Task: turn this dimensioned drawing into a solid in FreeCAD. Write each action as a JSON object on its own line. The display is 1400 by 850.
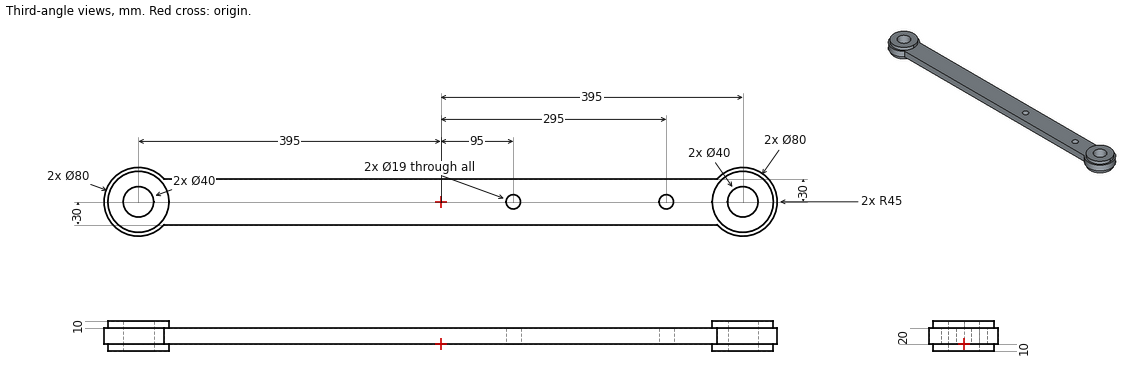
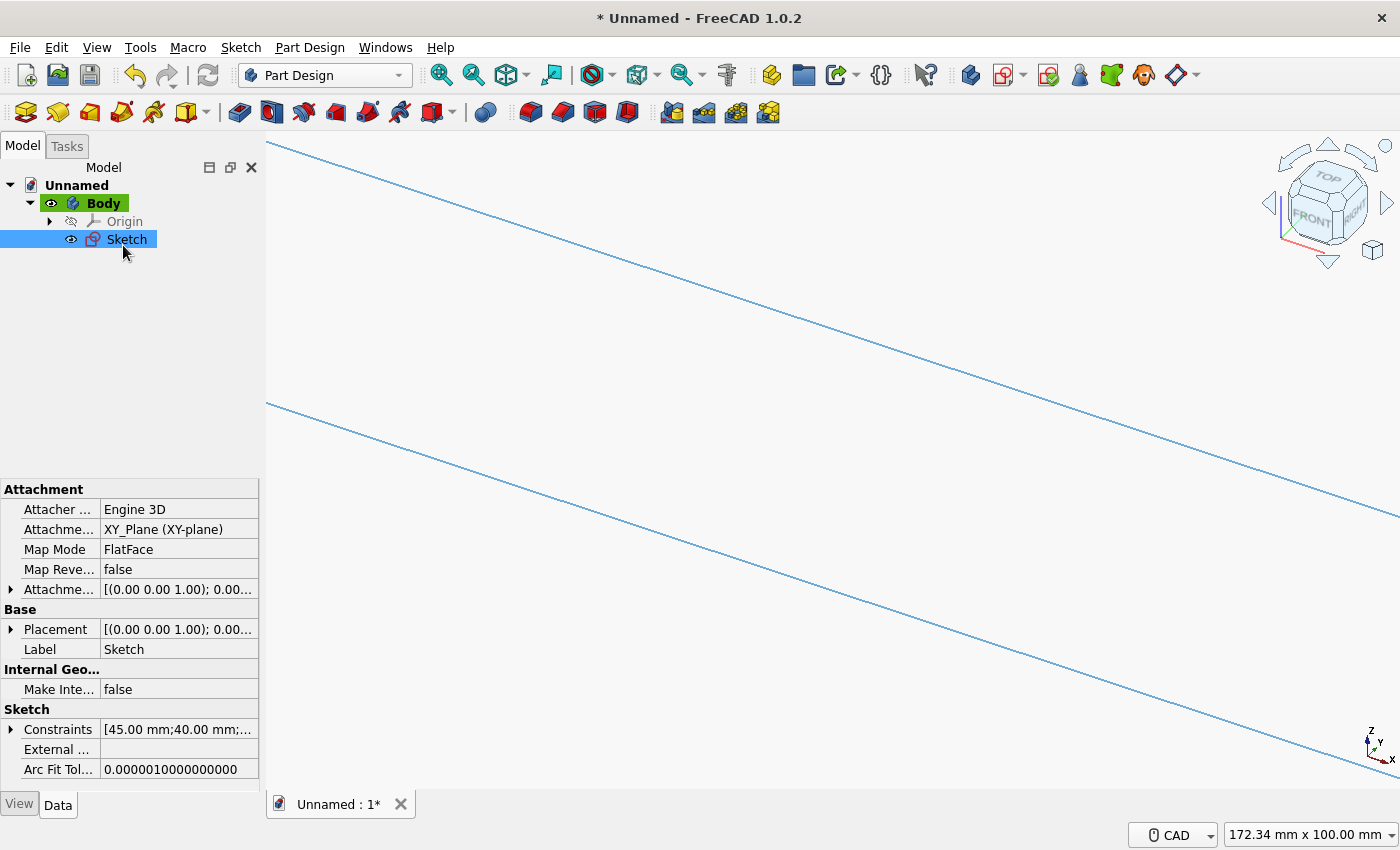
{"action": "left_click", "coordinate": [26, 112]}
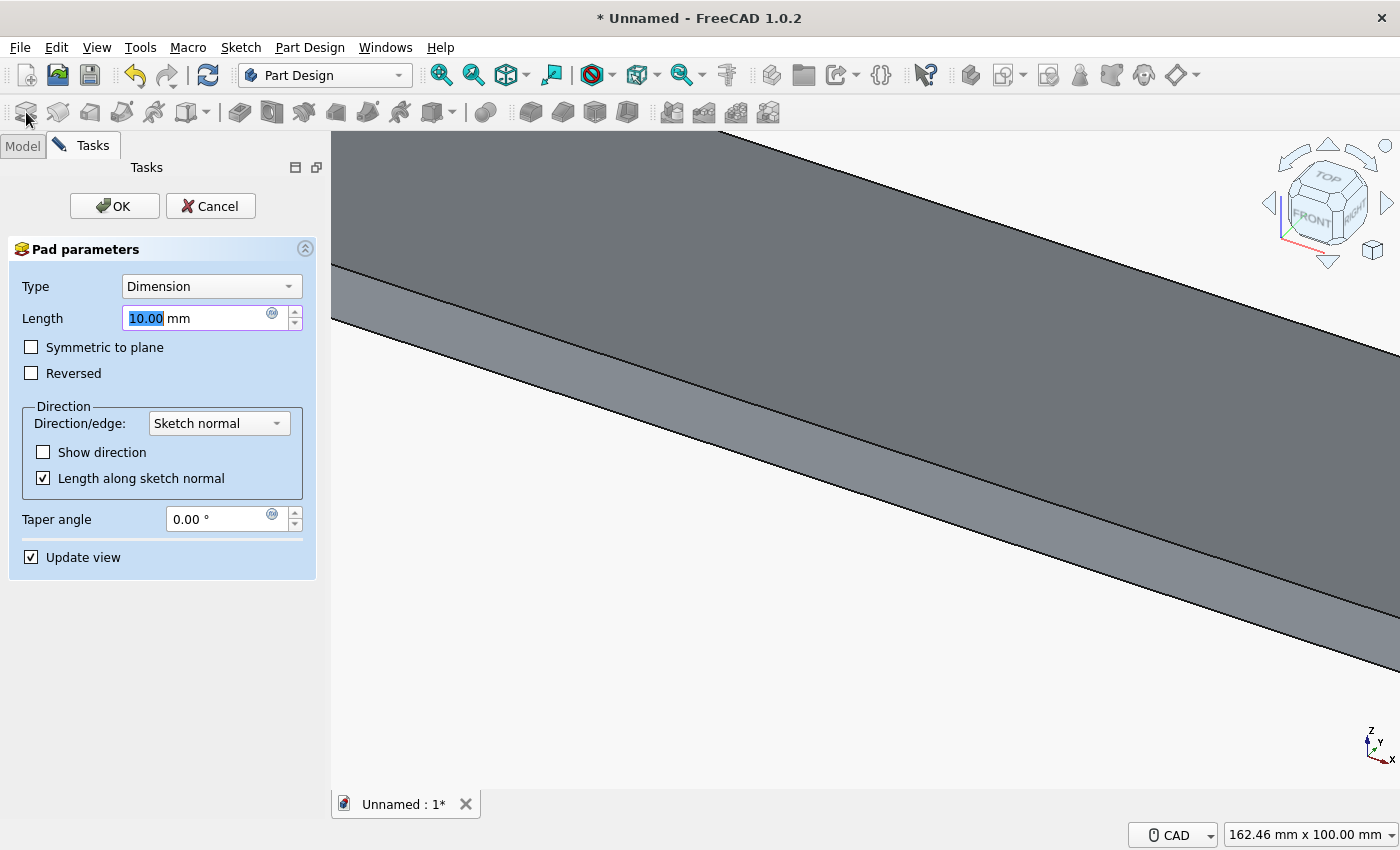
{"action": "type", "text": "20"}
{"action": "key", "text": "Tab"}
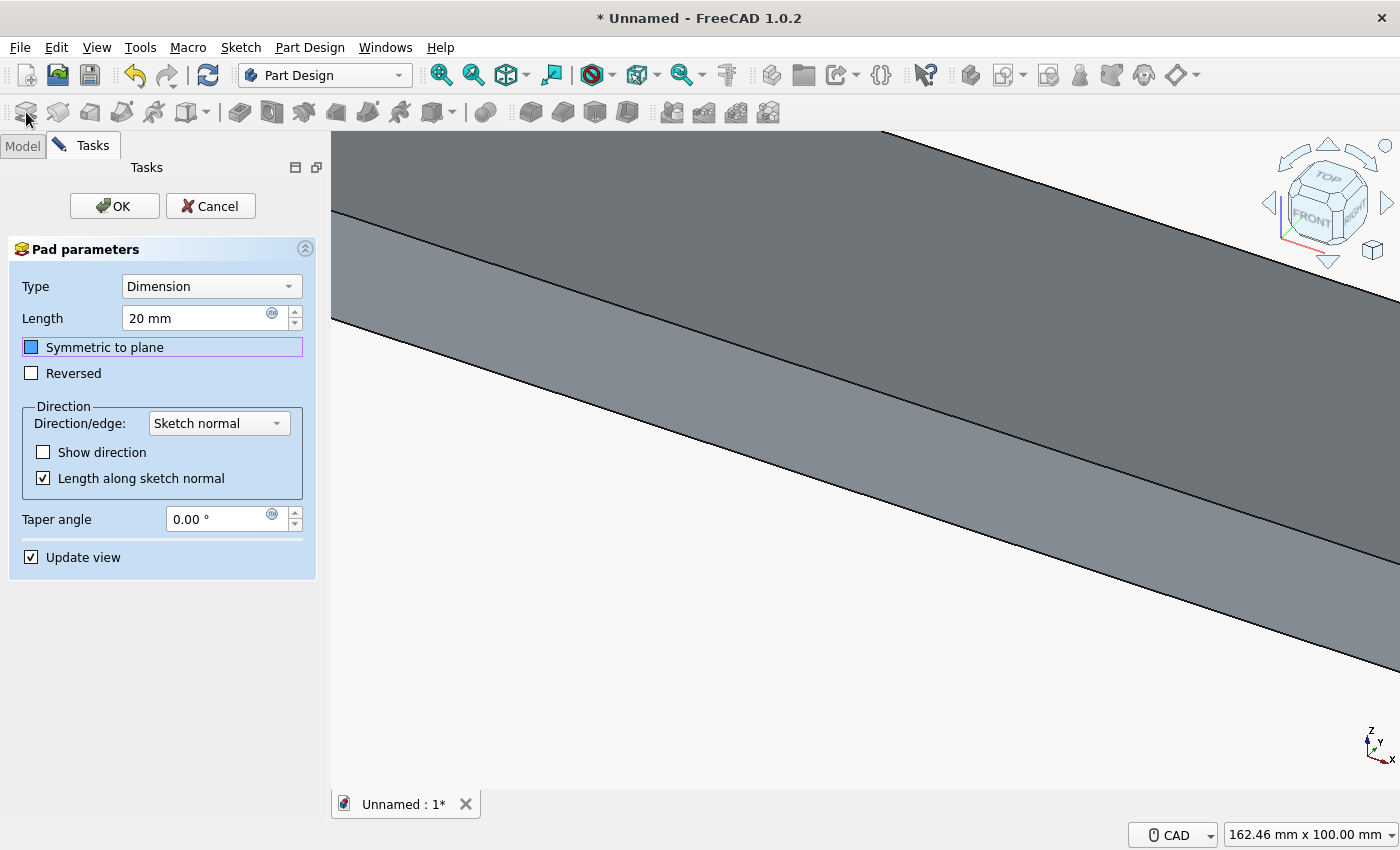
{"action": "left_click", "coordinate": [115, 206]}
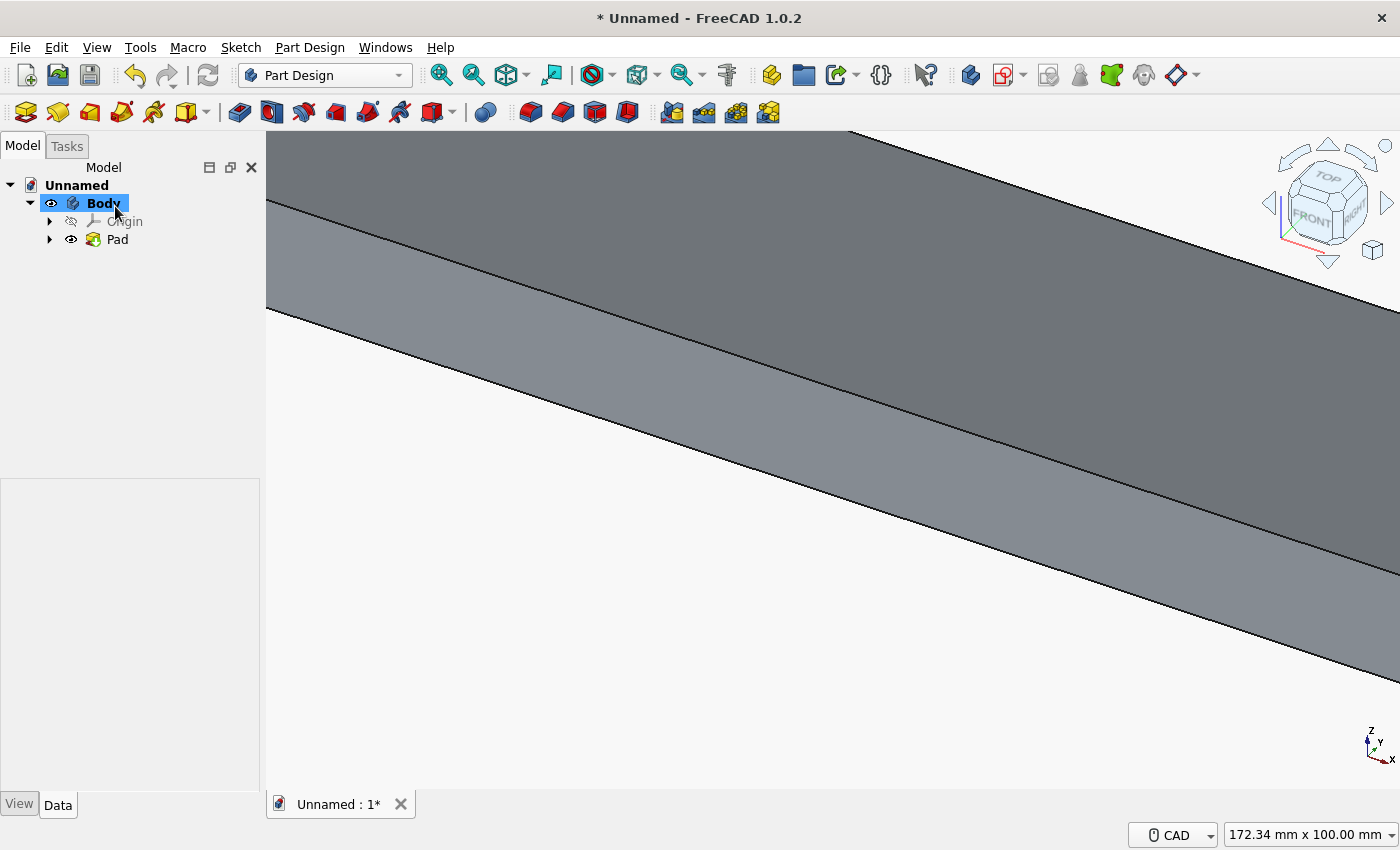
{"action": "left_click", "coordinate": [442, 76]}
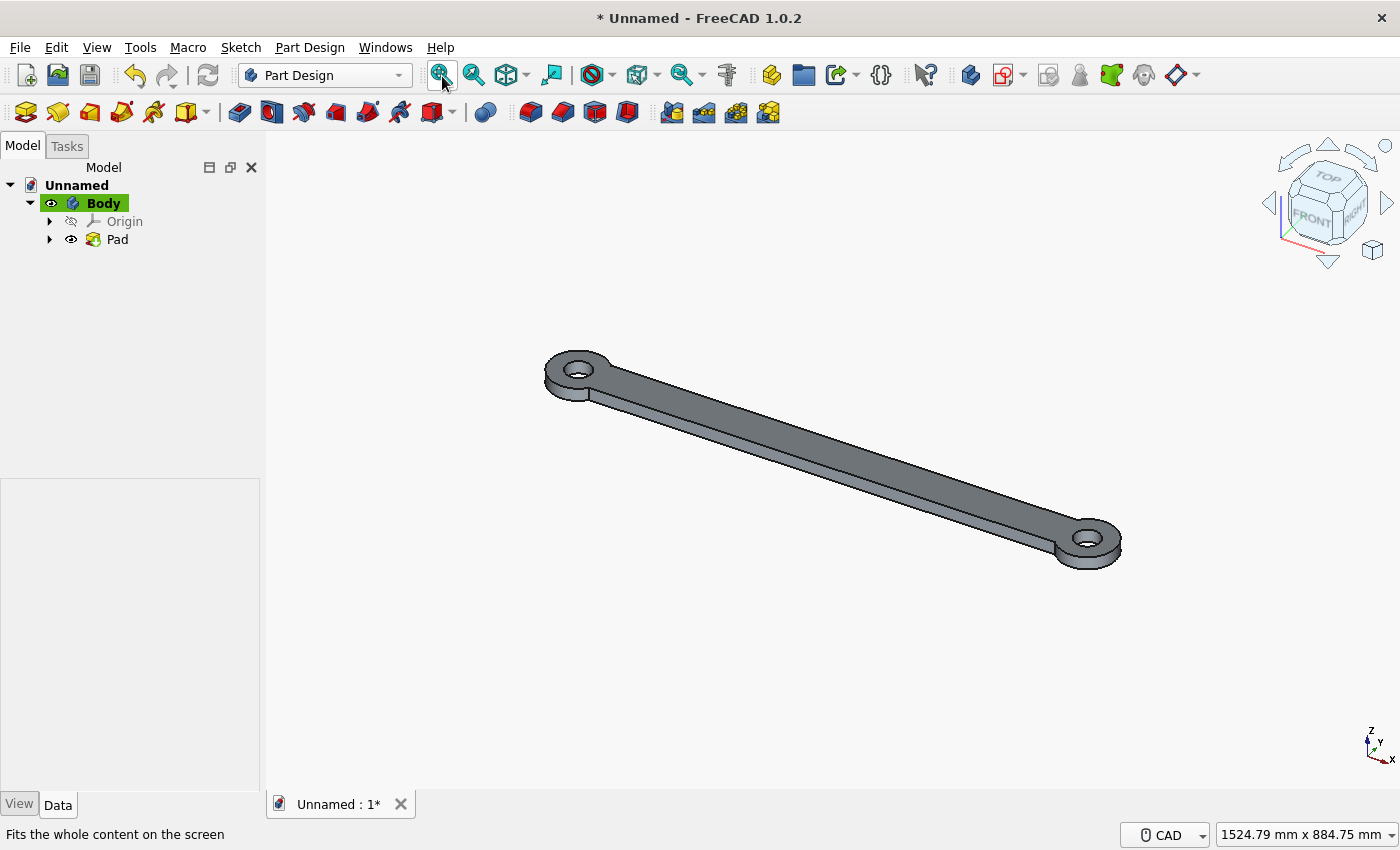
{"action": "left_click", "coordinate": [995, 507]}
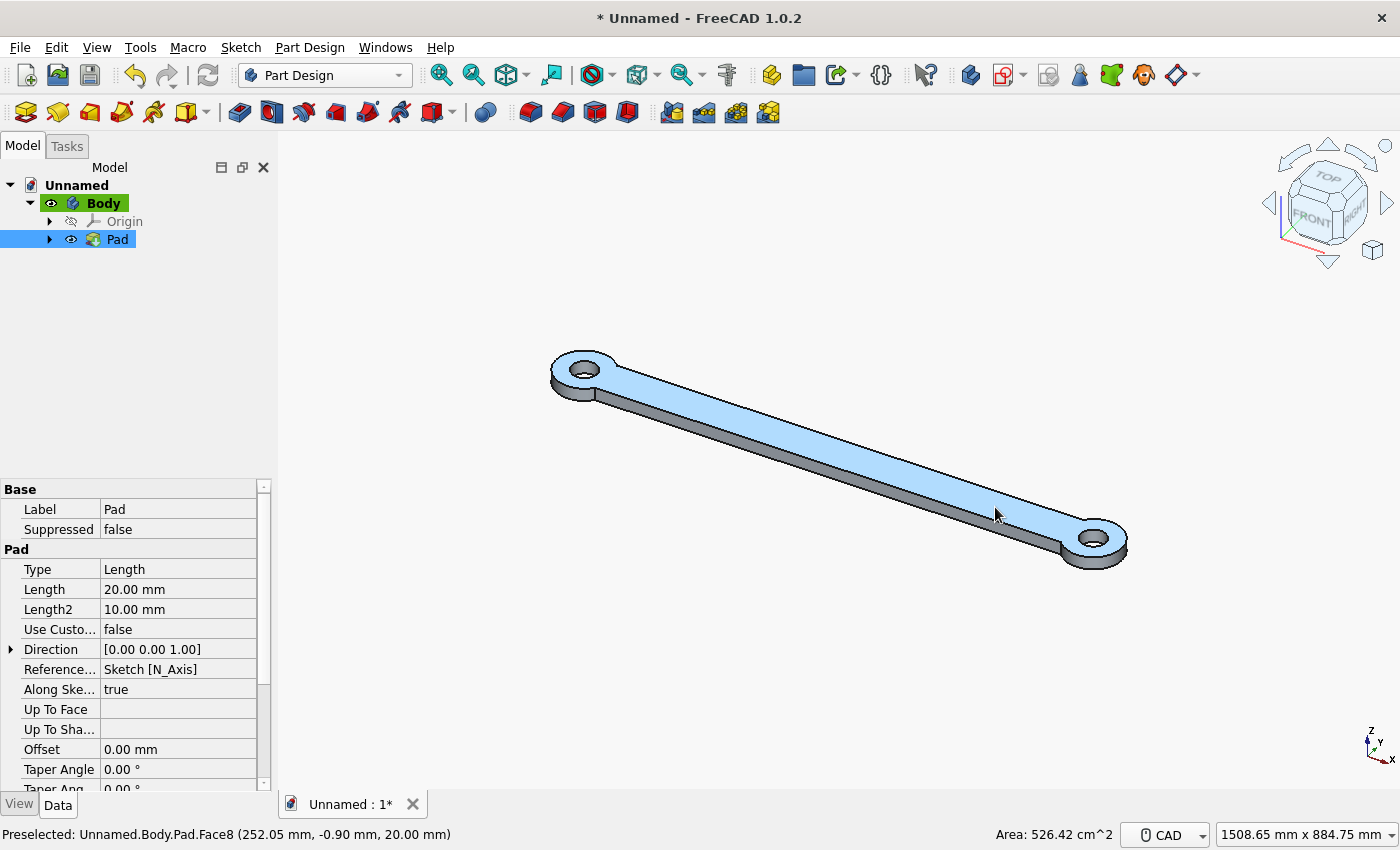
{"action": "left_click", "coordinate": [1004, 76]}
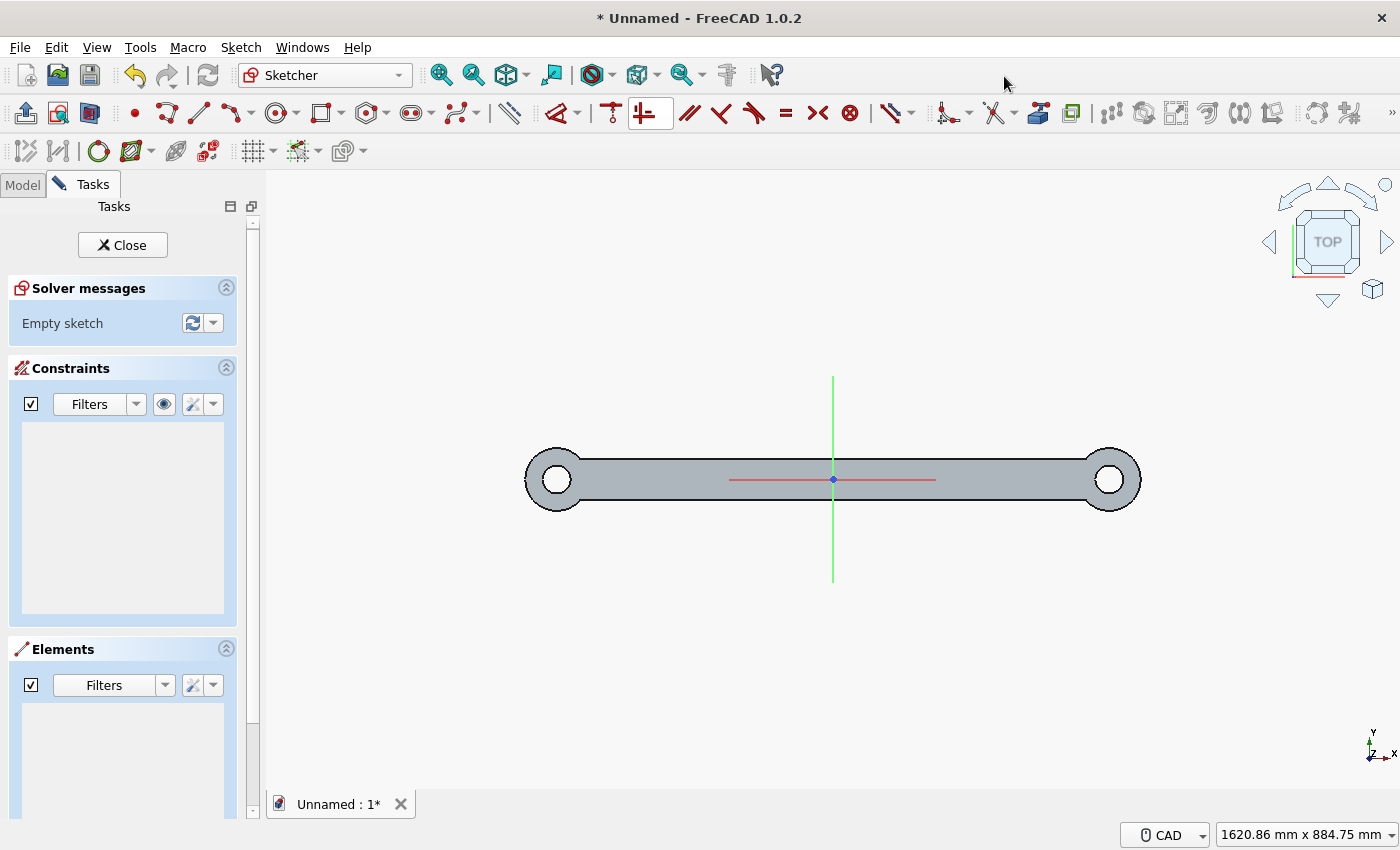
{"action": "left_click", "coordinate": [276, 114]}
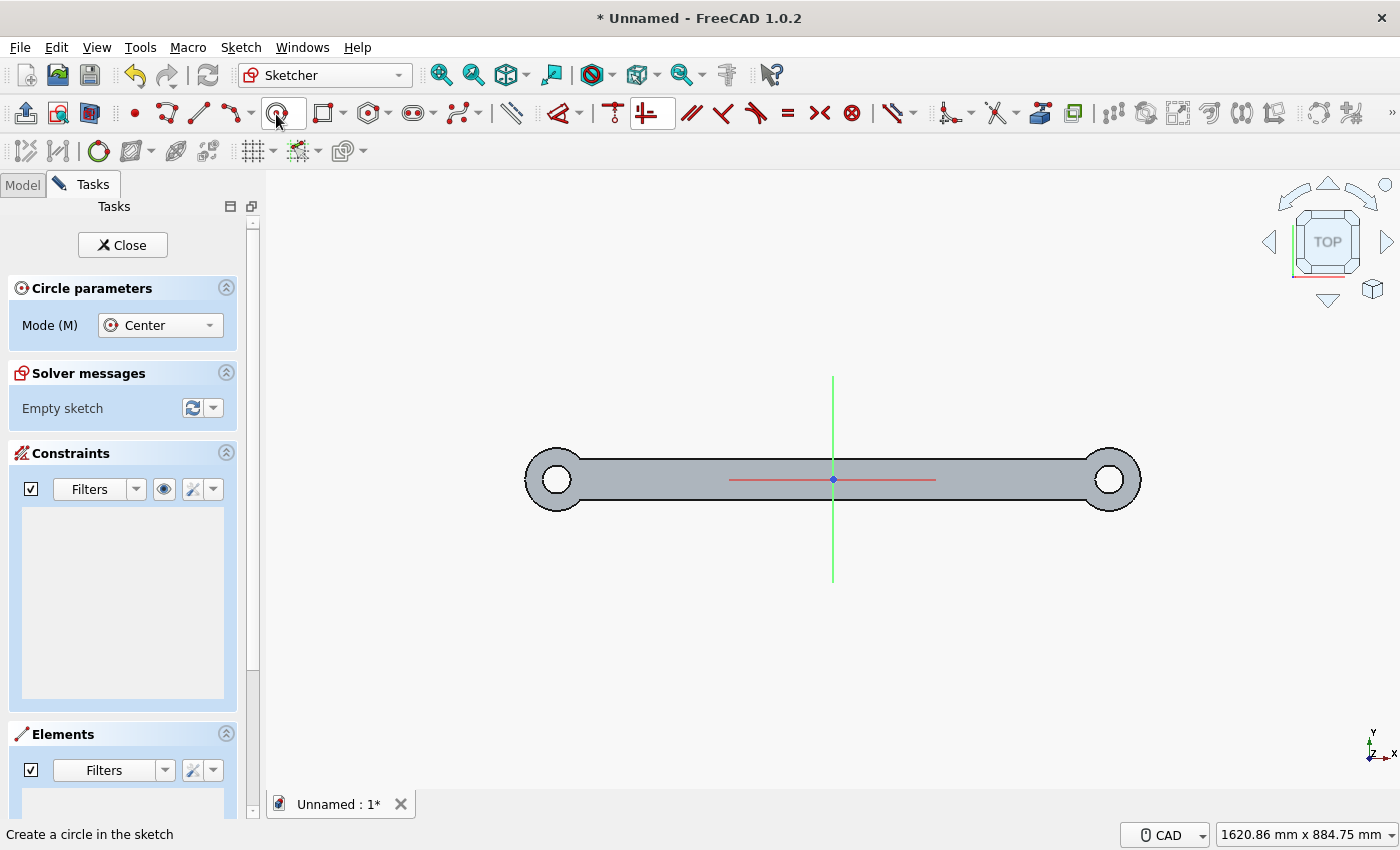
{"action": "left_click", "coordinate": [557, 480]}
{"action": "left_click", "coordinate": [576, 460]}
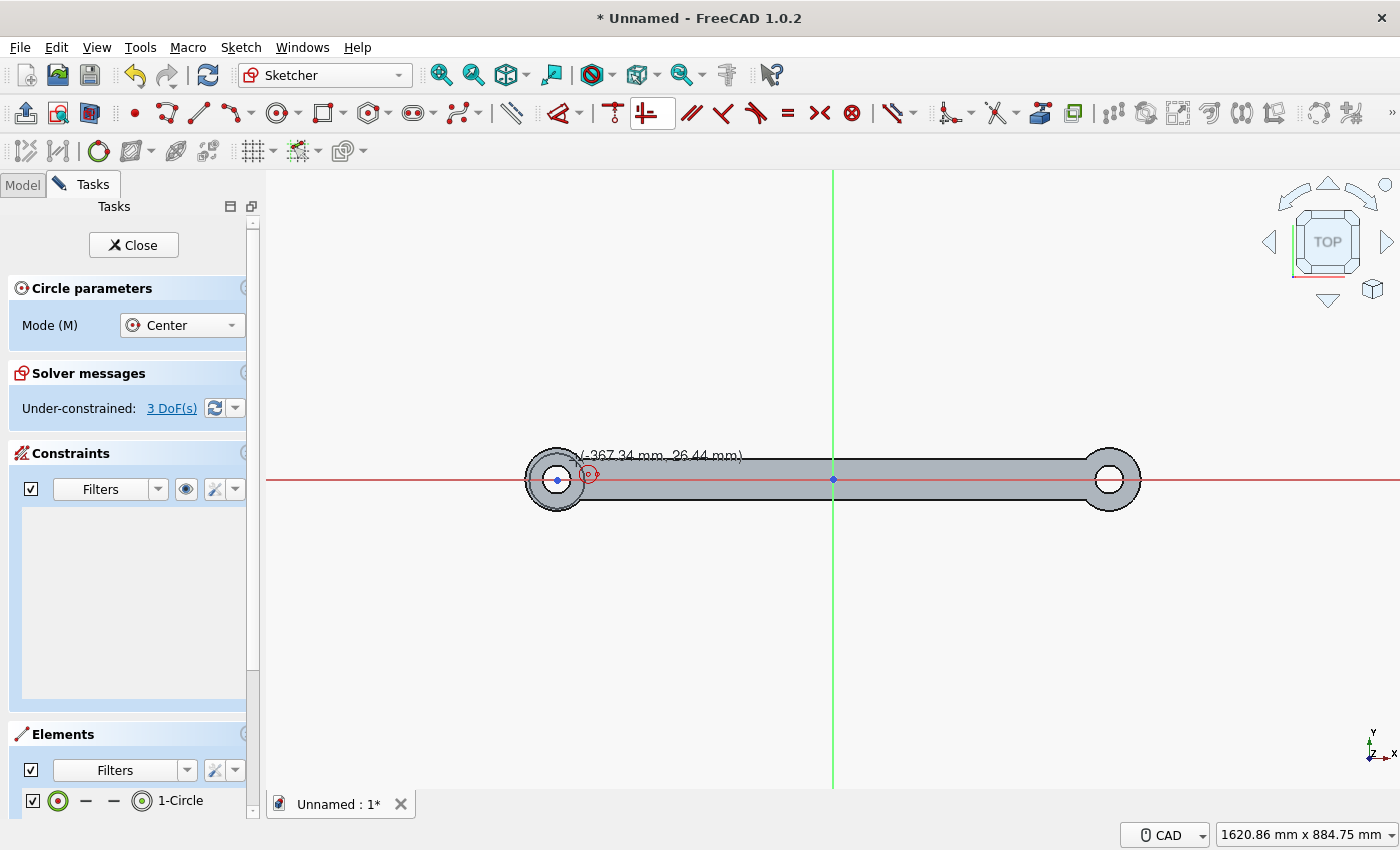
{"action": "left_click", "coordinate": [1109, 480]}
{"action": "left_click", "coordinate": [1129, 460]}